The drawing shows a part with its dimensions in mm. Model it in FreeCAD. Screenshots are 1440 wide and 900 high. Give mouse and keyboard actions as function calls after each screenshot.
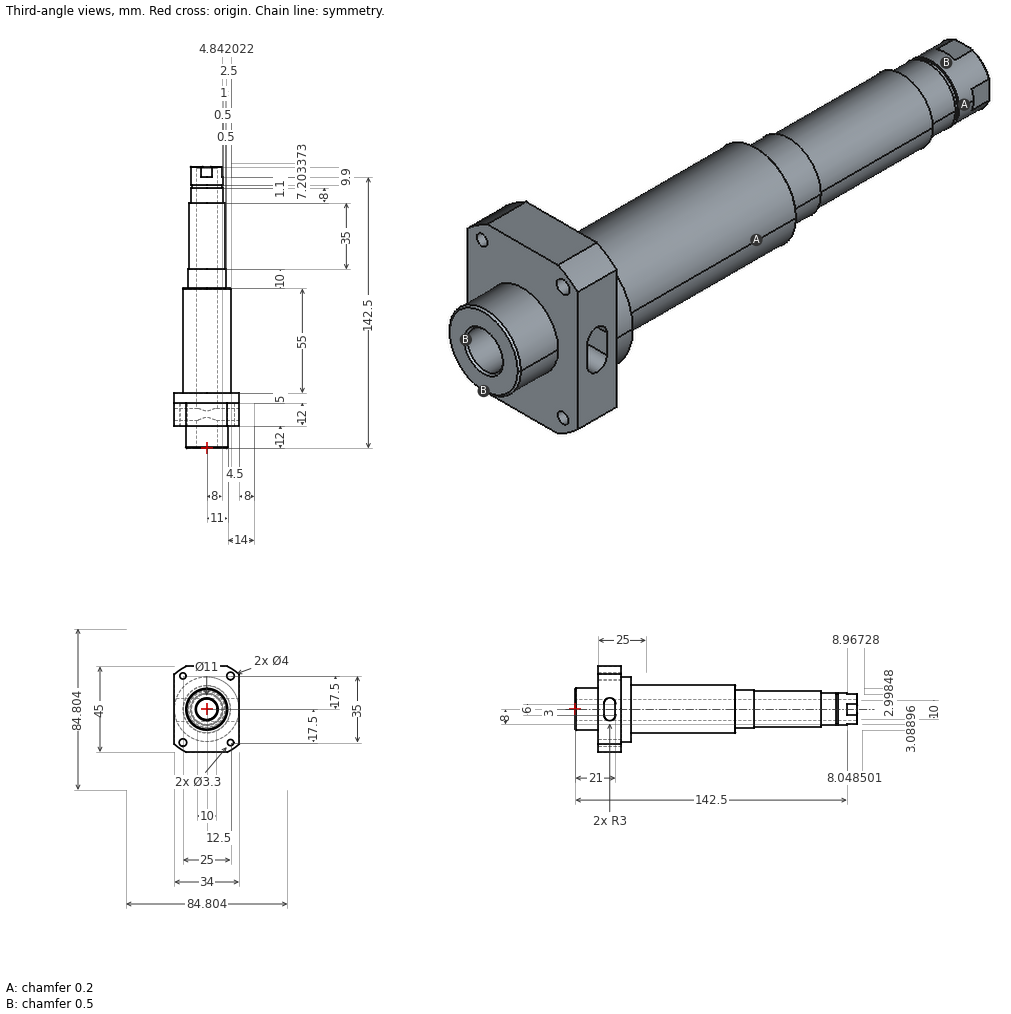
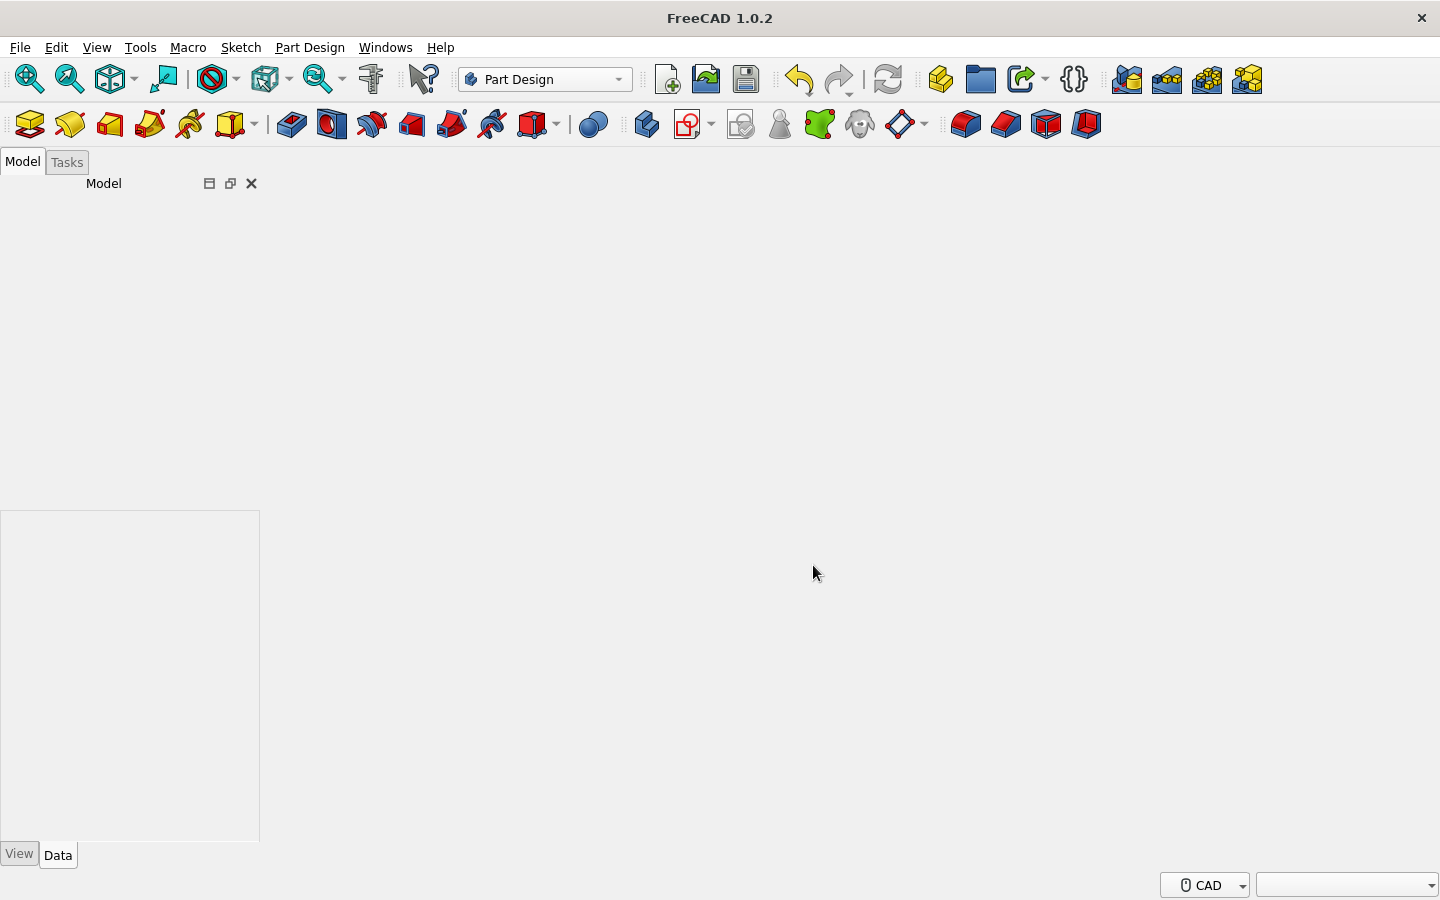
click(666, 80)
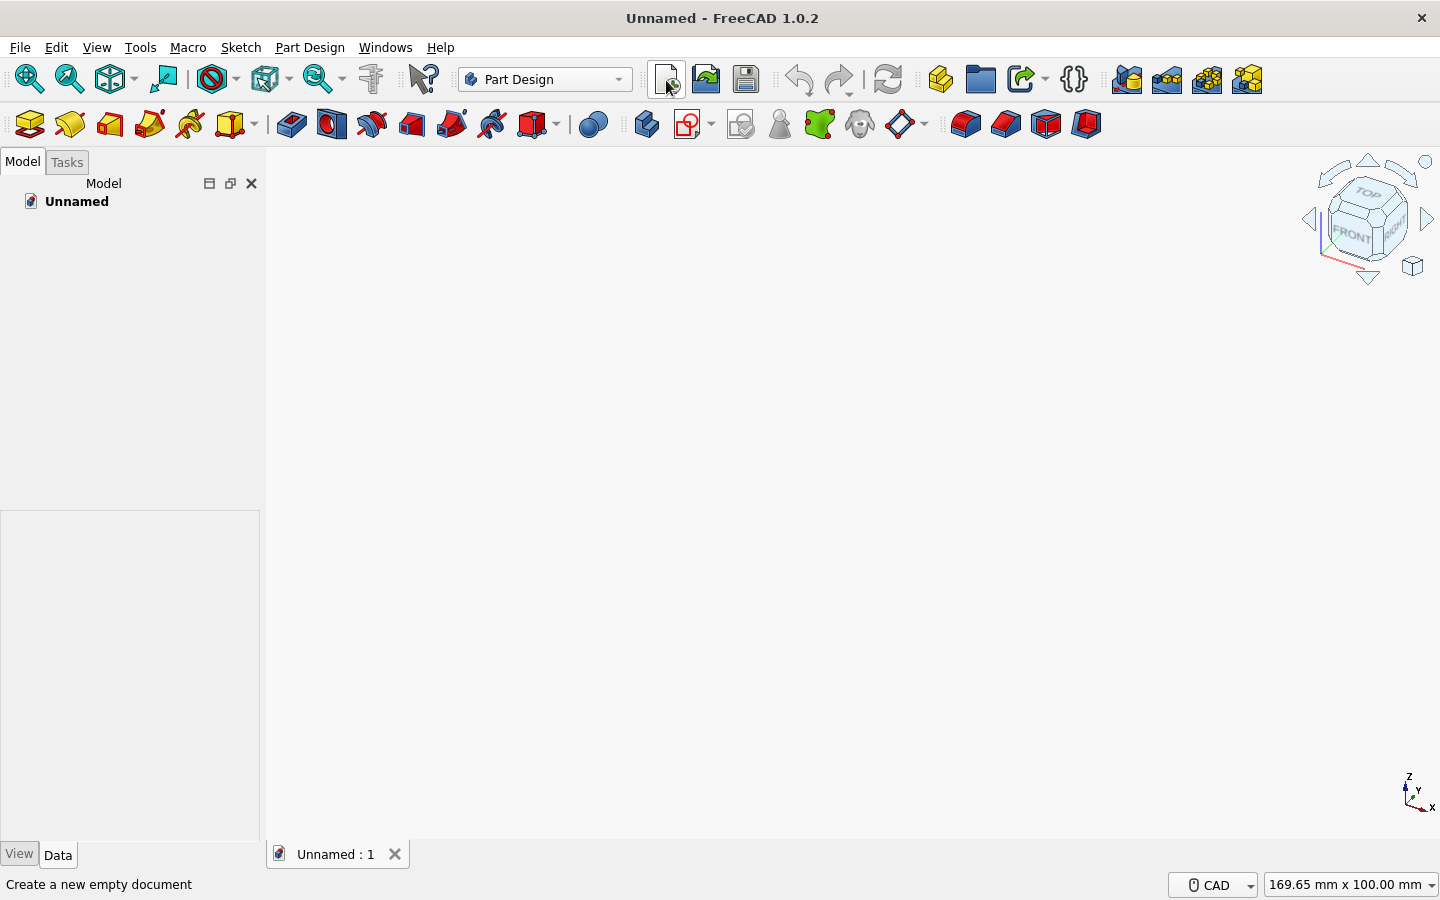
click(688, 124)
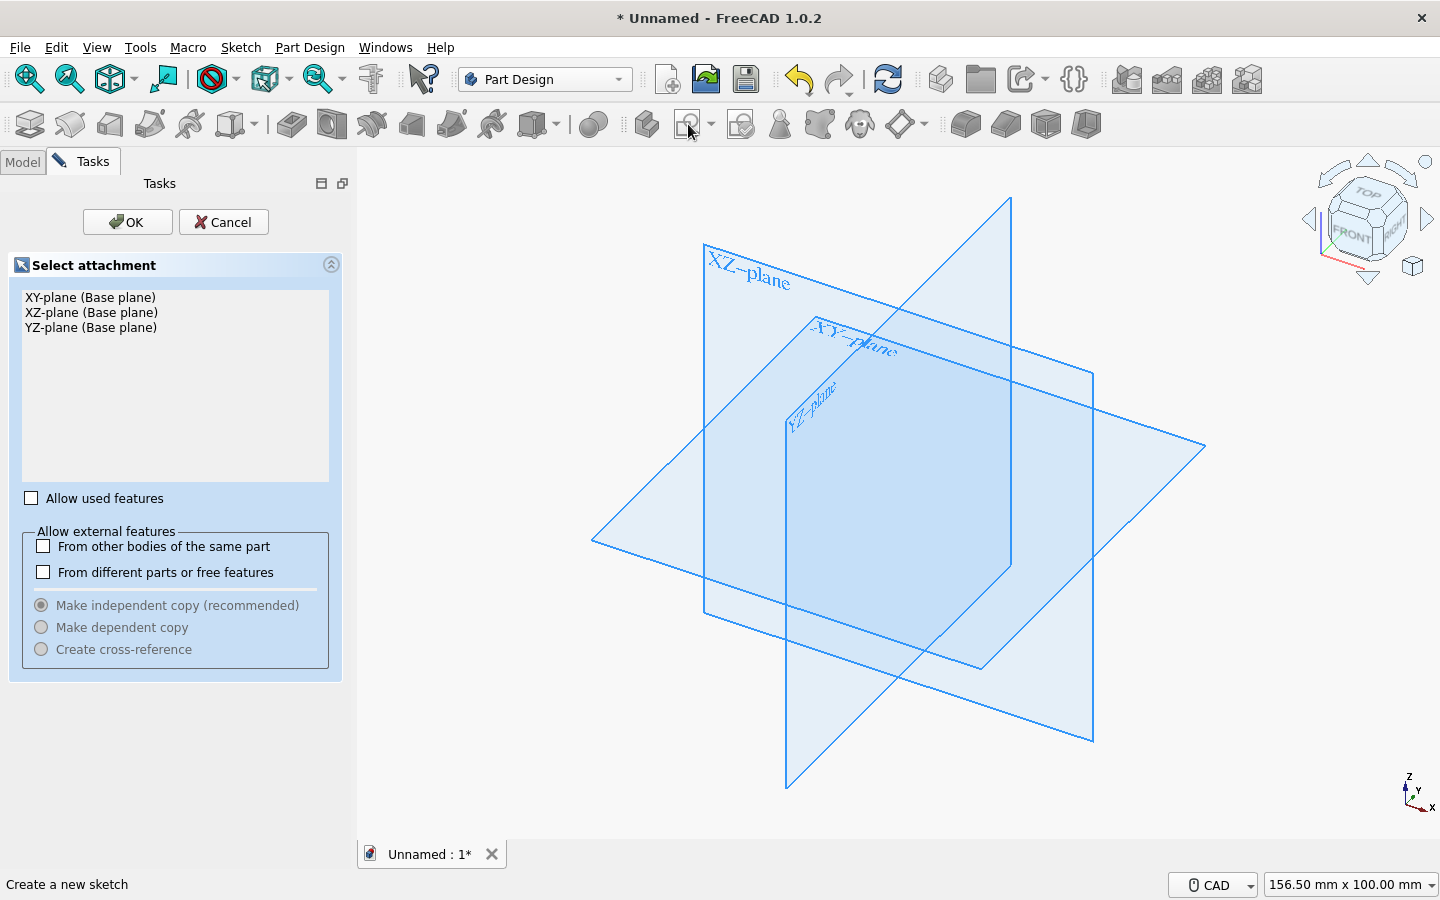
click(82, 298)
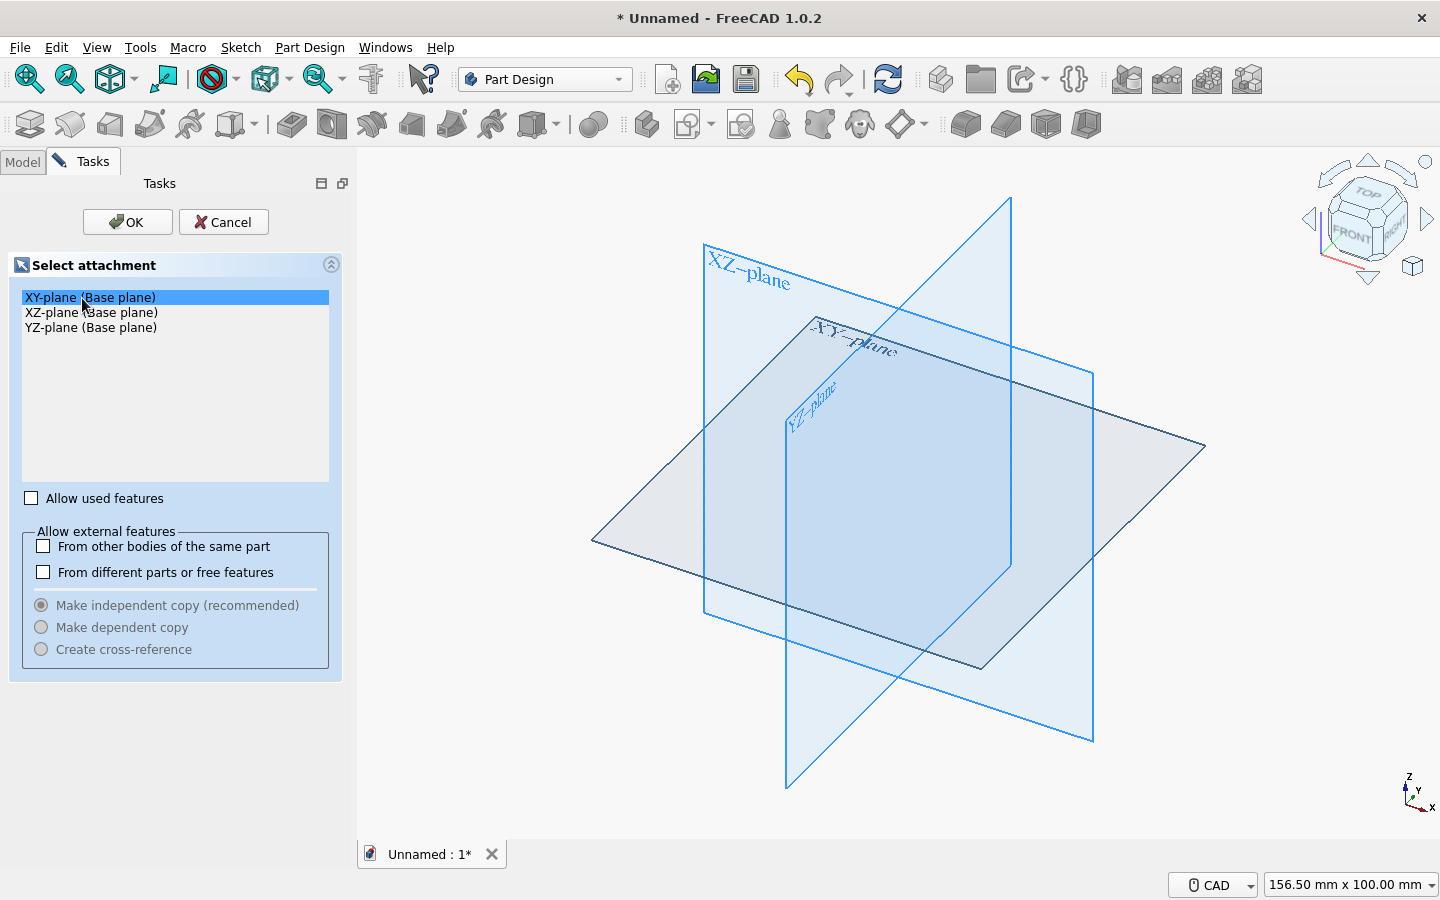
click(128, 222)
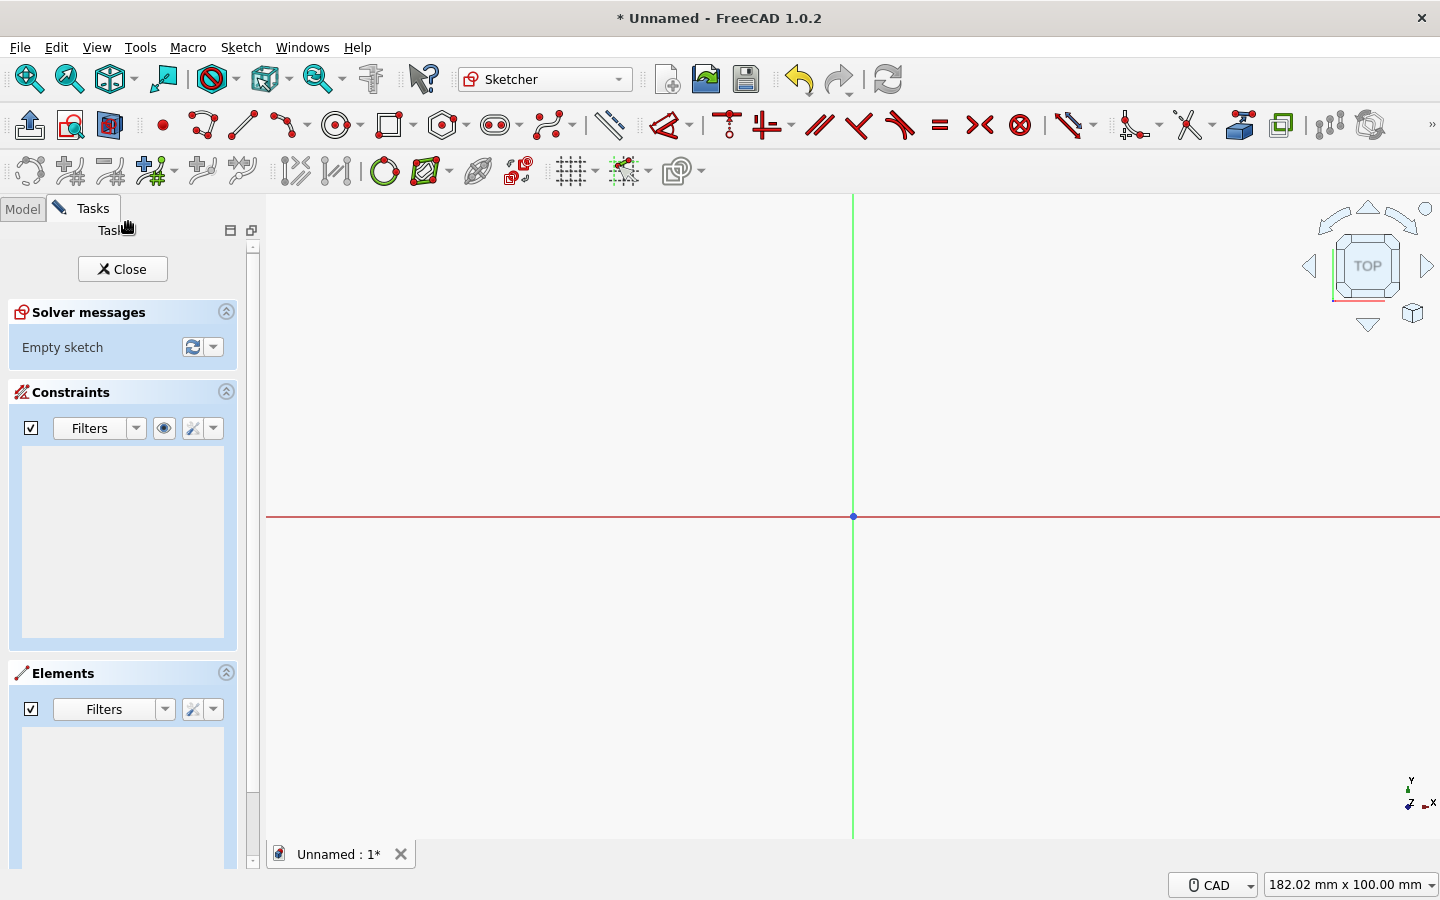
scroll(663, 811, down, 4)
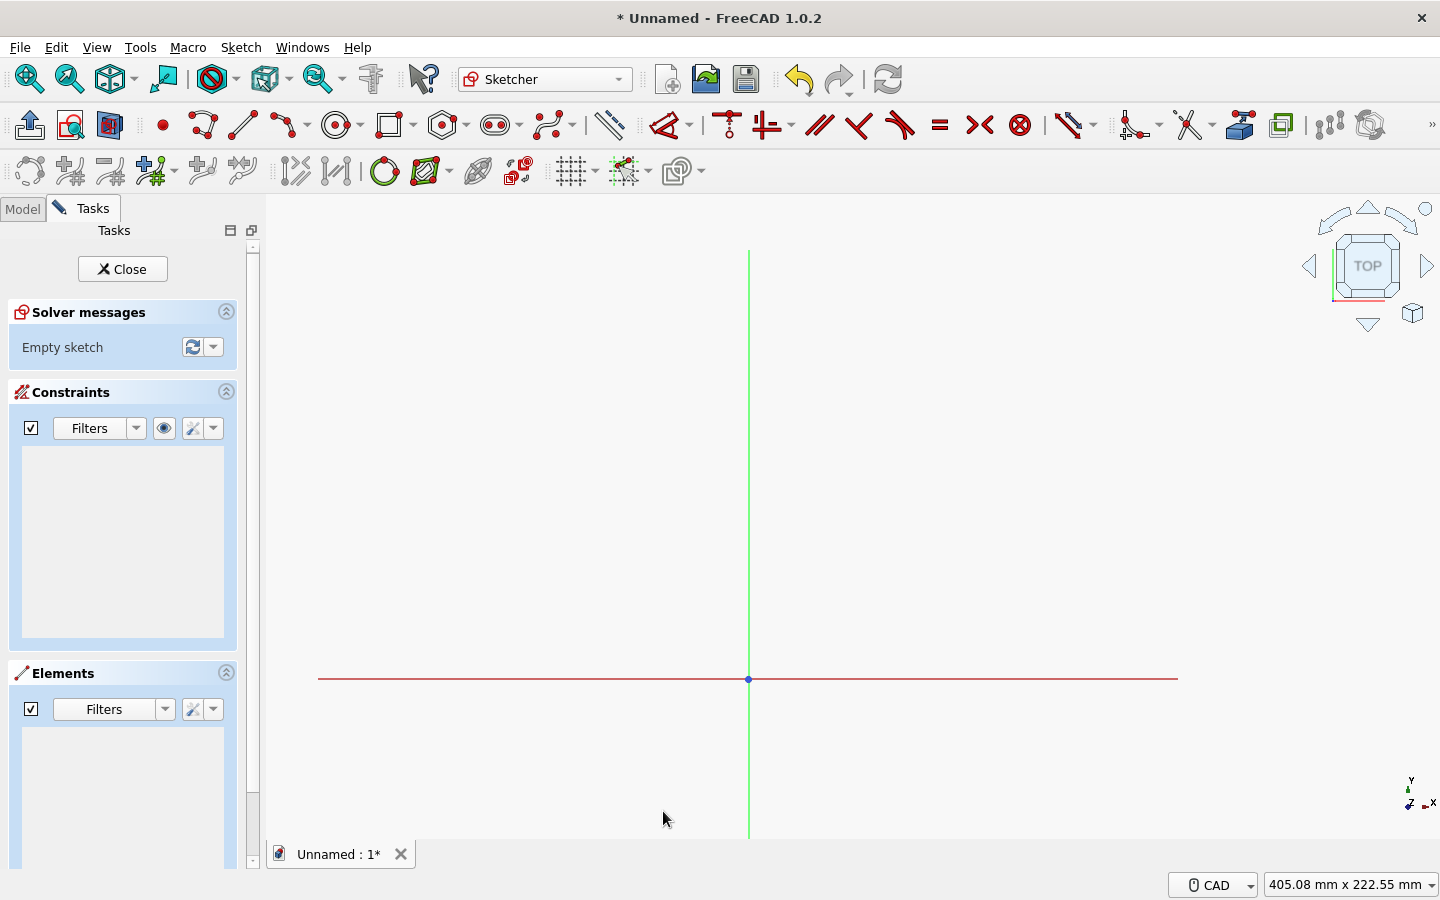
click(204, 126)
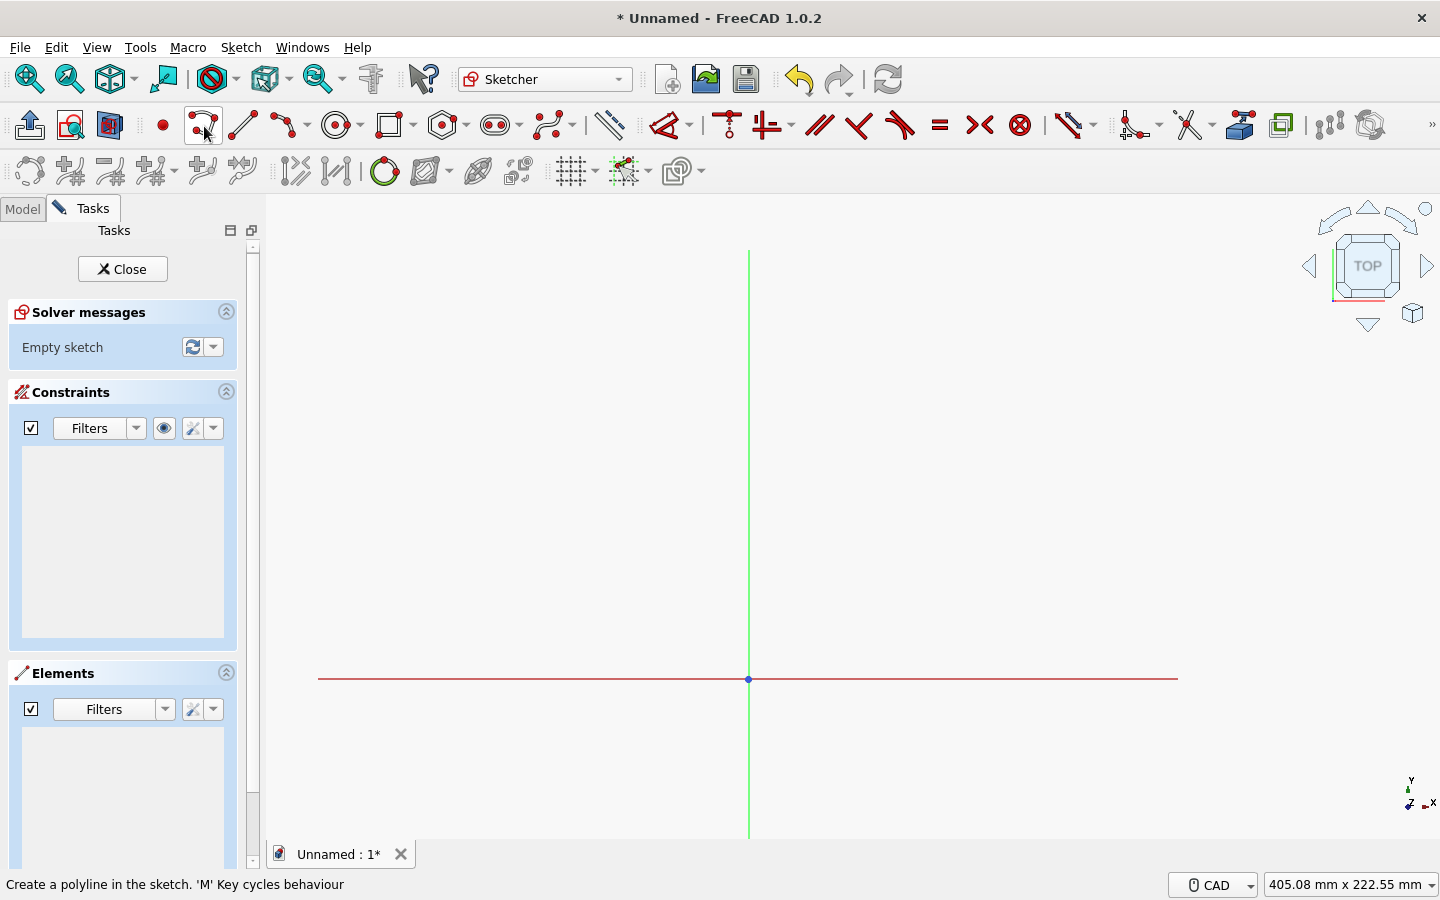
click(749, 679)
click(780, 670)
click(780, 644)
click(821, 644)
click(821, 610)
click(798, 610)
click(798, 595)
click(785, 595)
click(785, 436)